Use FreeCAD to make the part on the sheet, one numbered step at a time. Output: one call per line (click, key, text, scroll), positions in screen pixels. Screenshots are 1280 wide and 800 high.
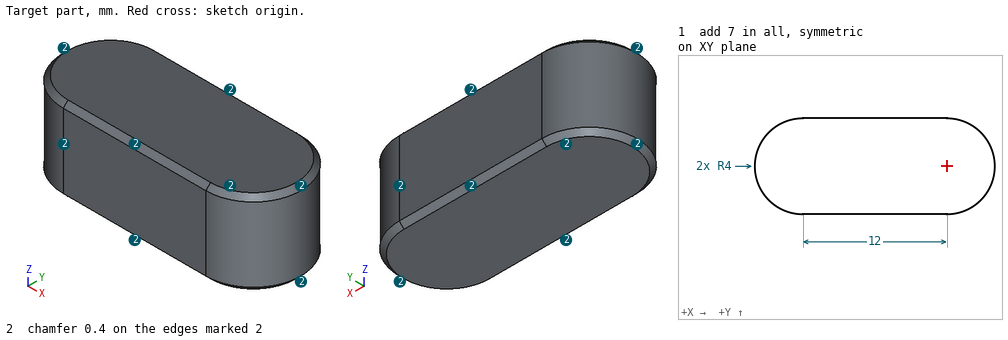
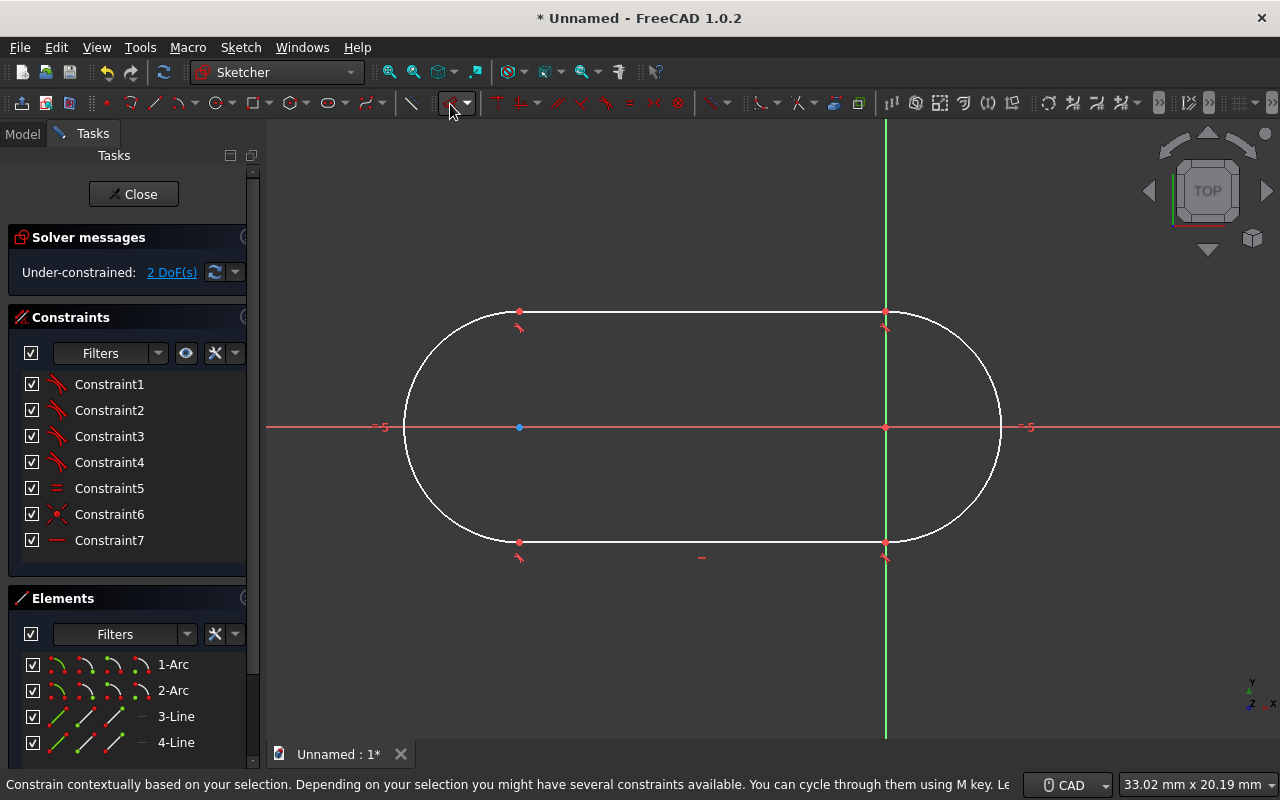
click(979, 495)
click(1005, 514)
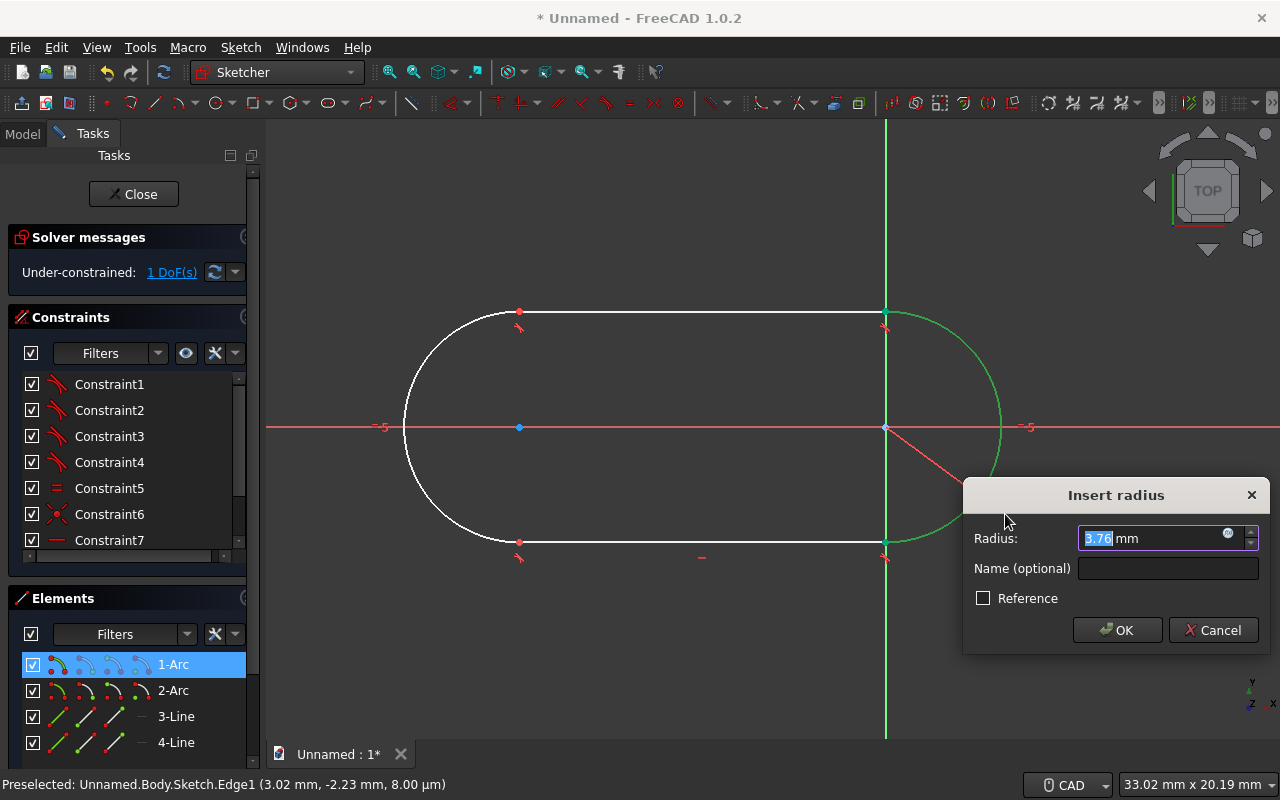
text(4)
key(Return)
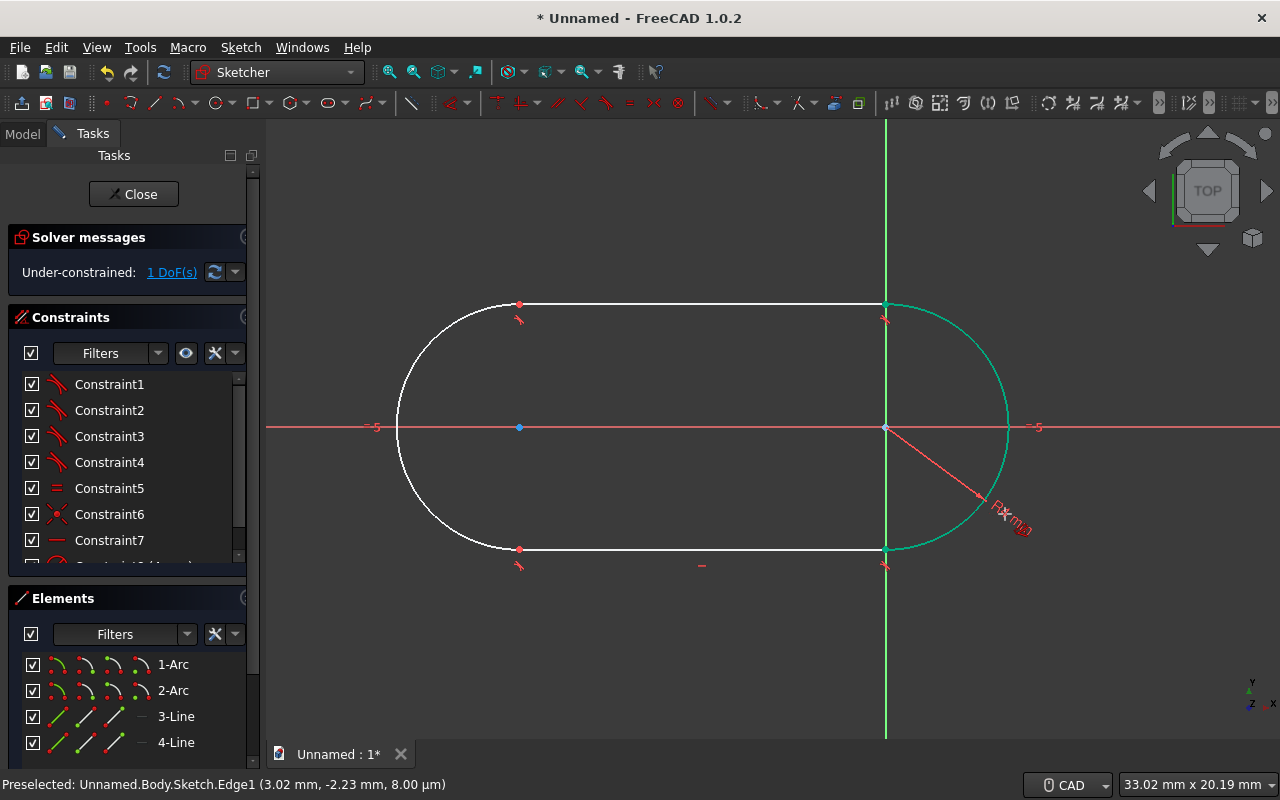
click(776, 550)
click(703, 584)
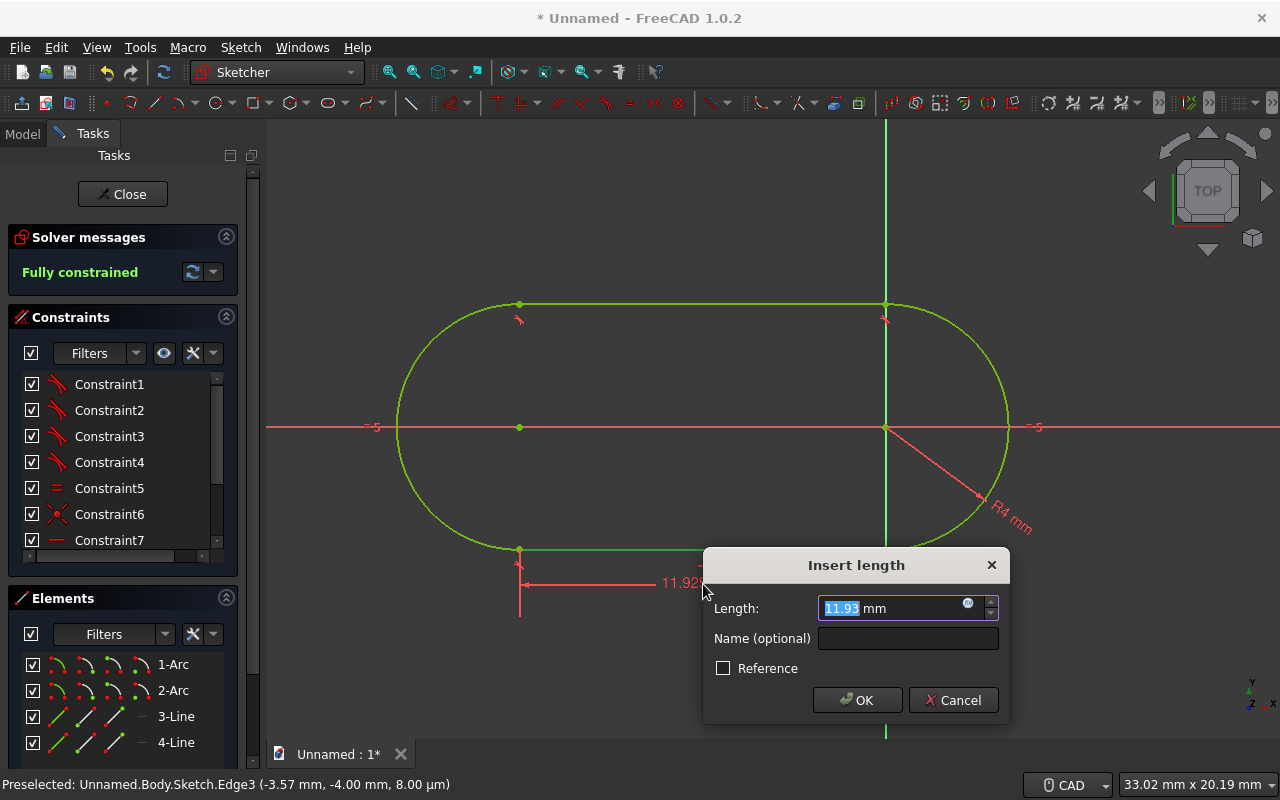
text(12)
key(Return)
key(Escape)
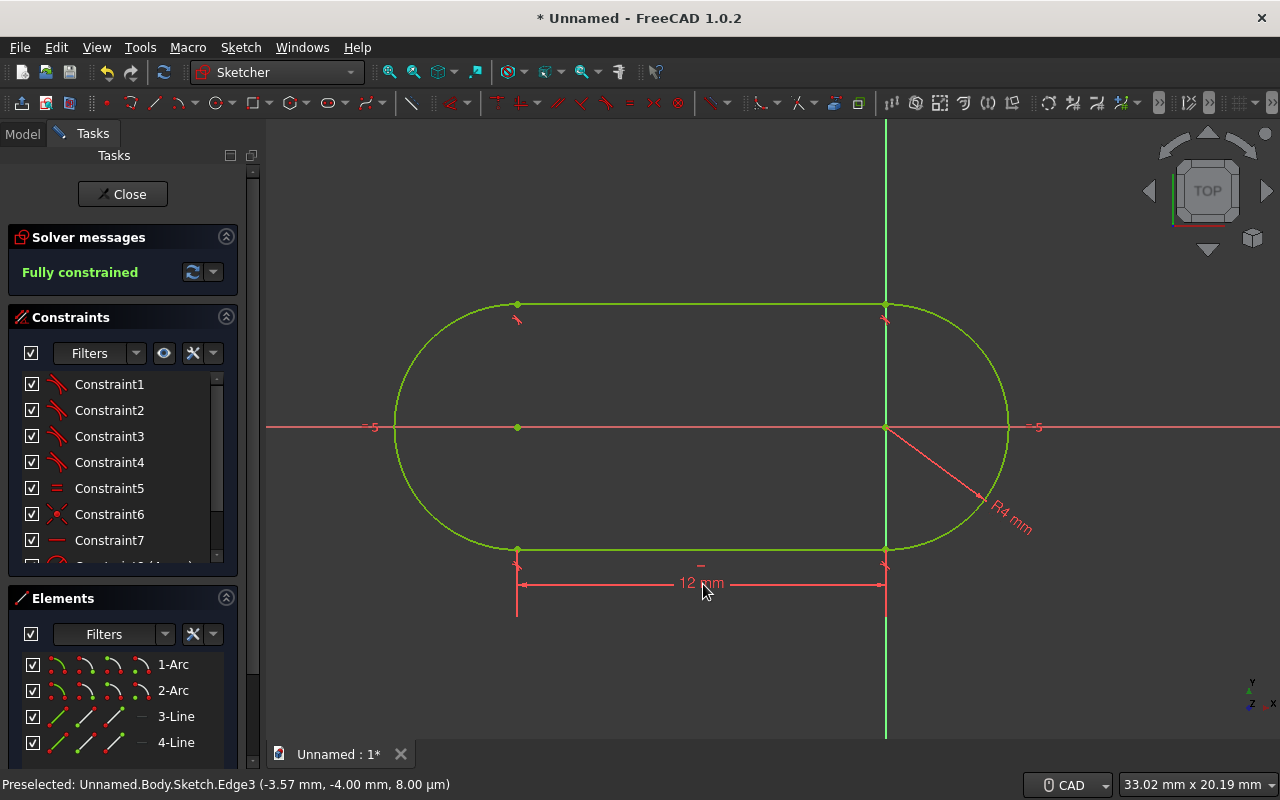
click(123, 194)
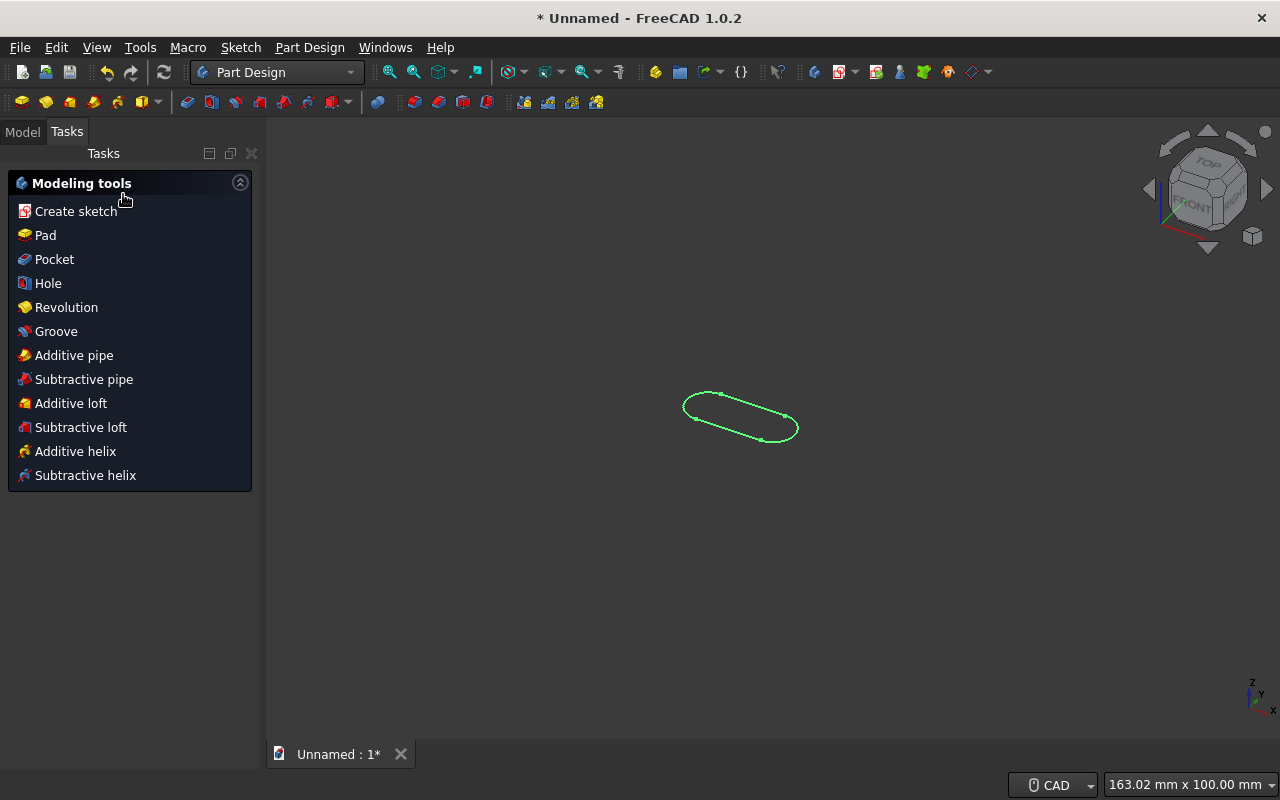
click(22, 102)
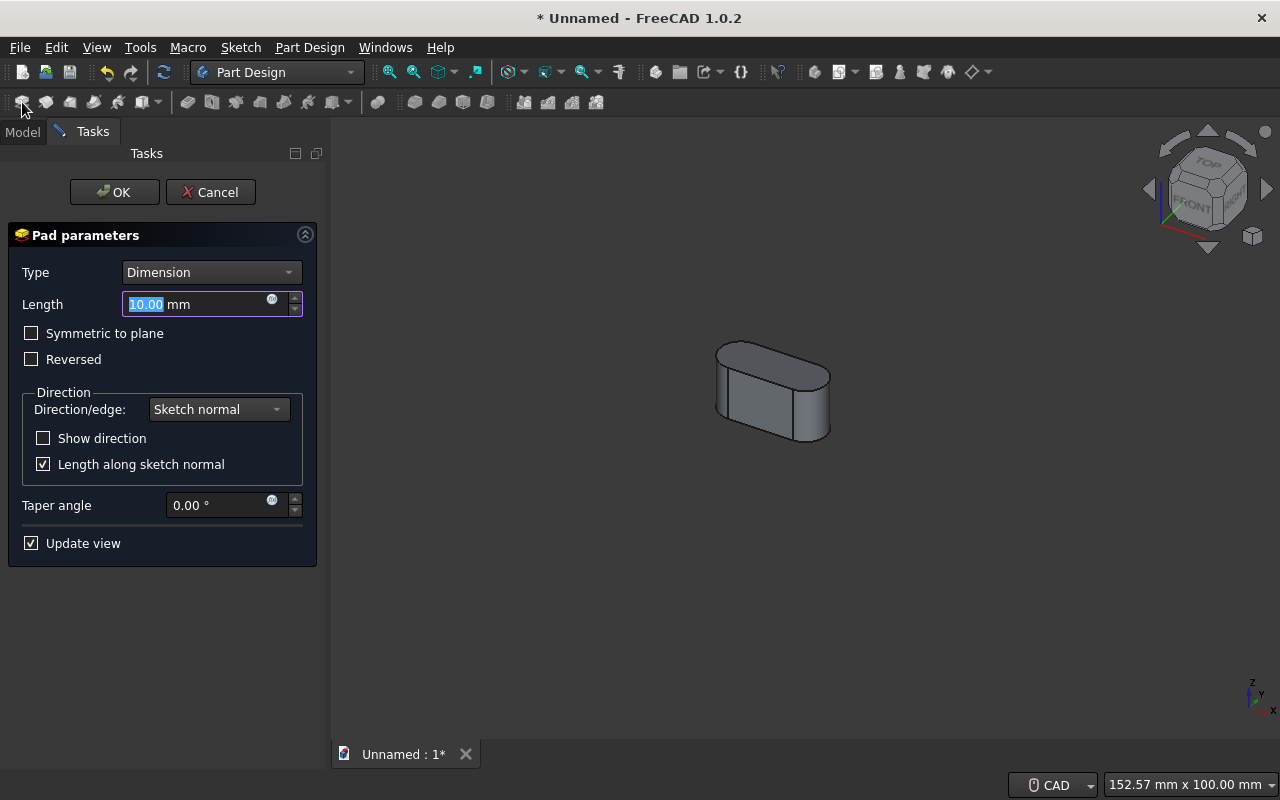
text(7)
key(Tab)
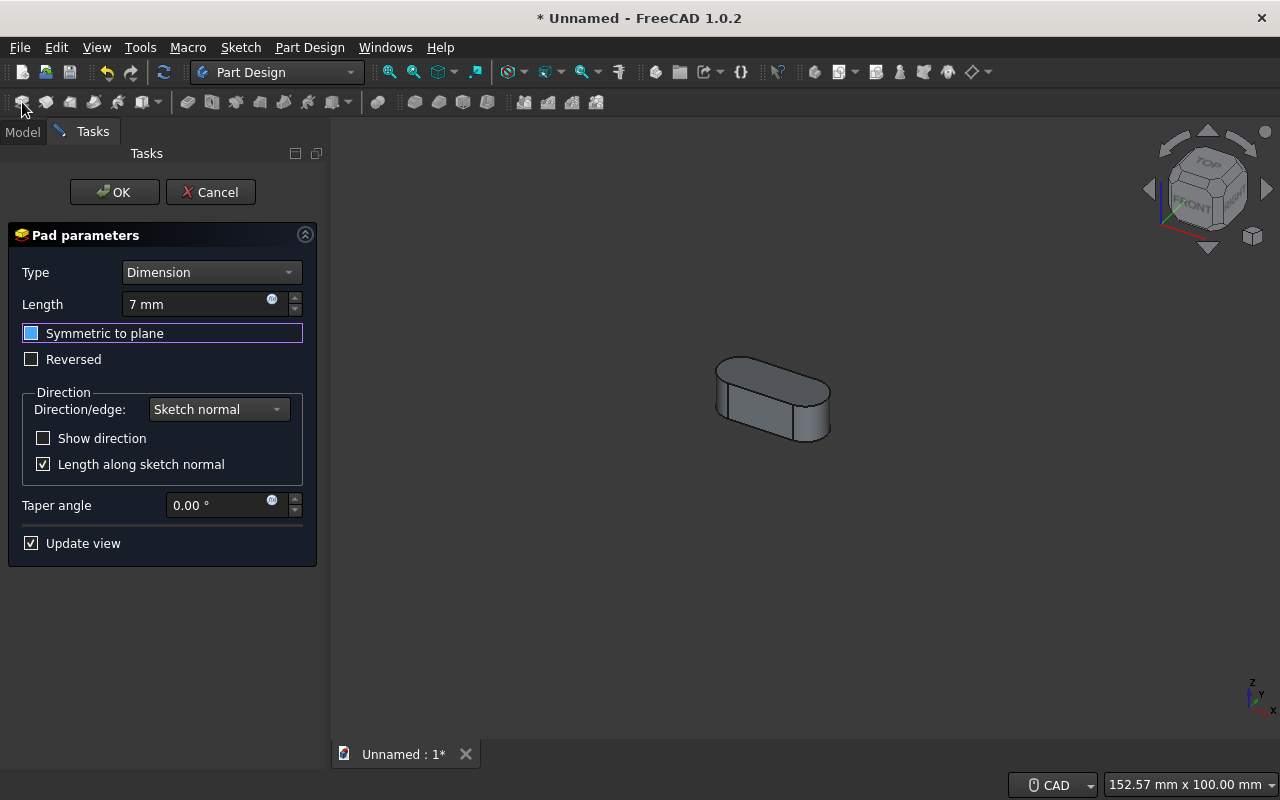
click(30, 333)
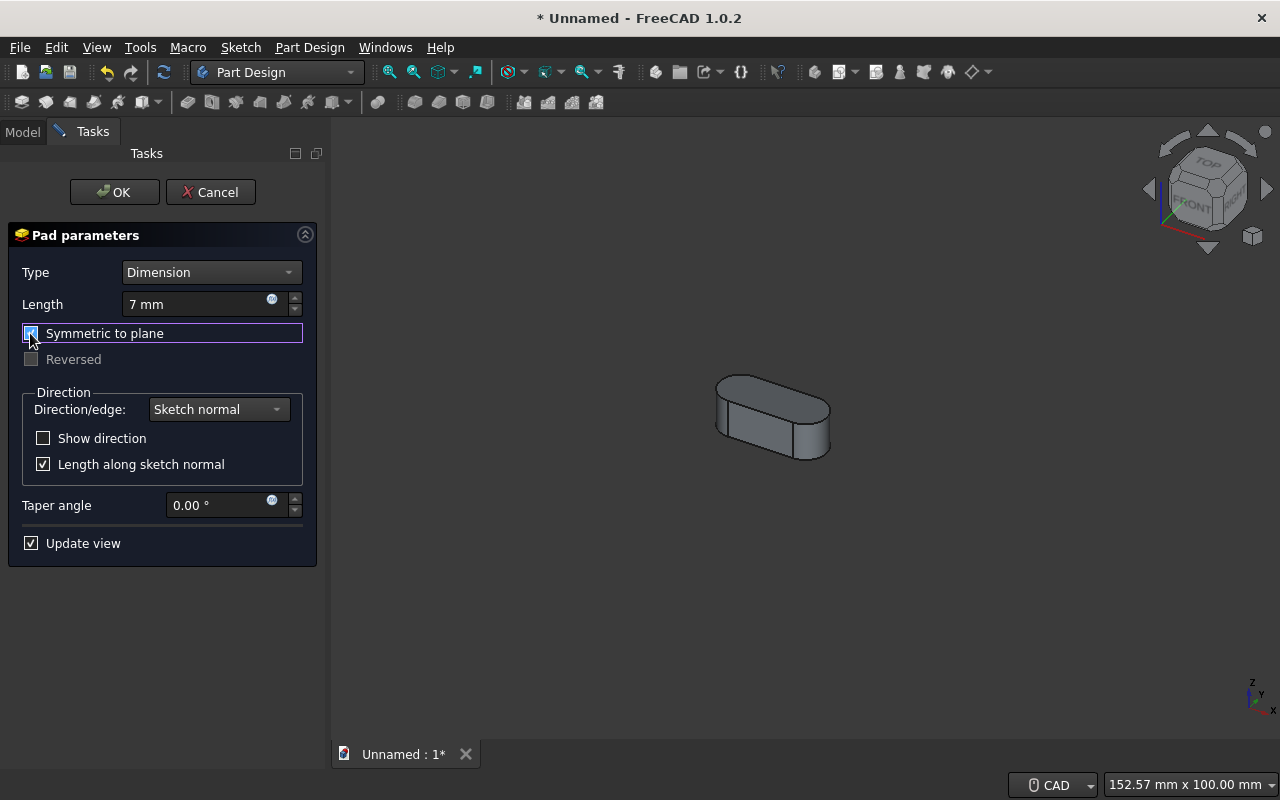
click(115, 192)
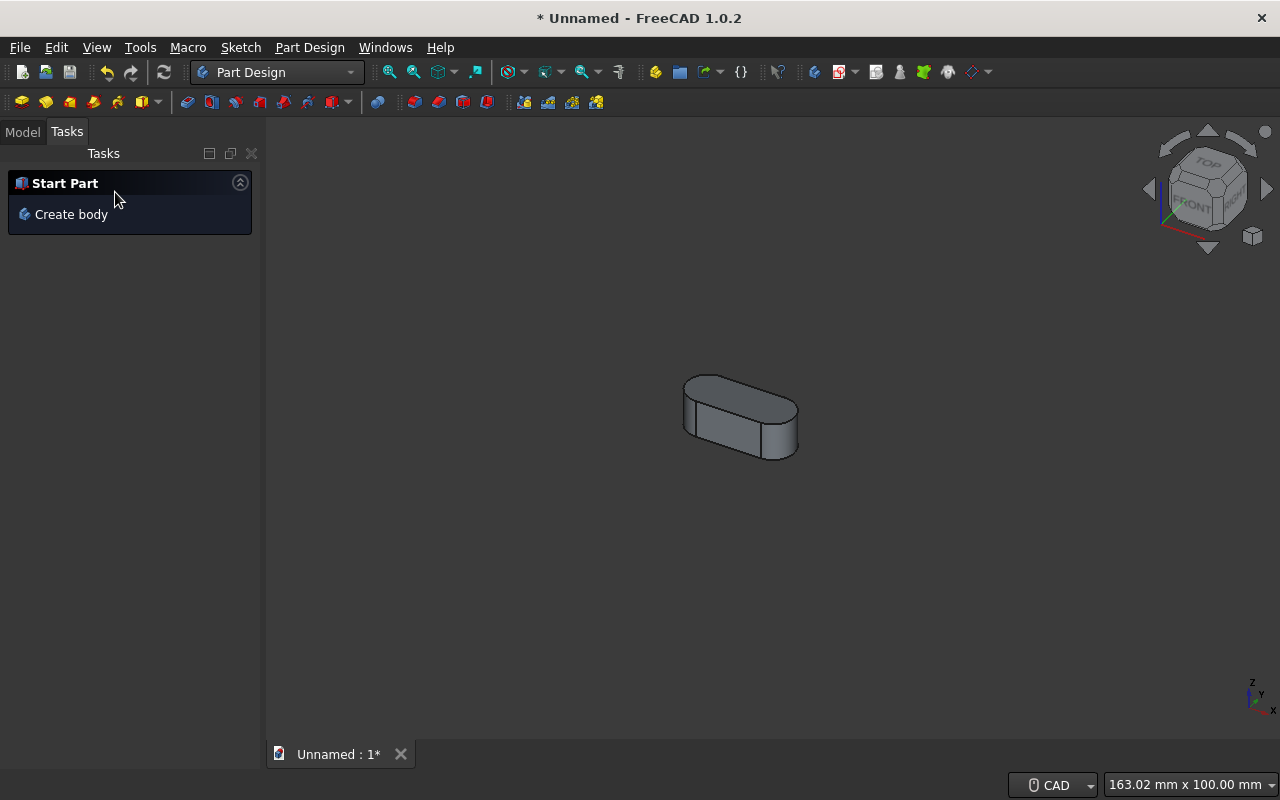
click(390, 72)